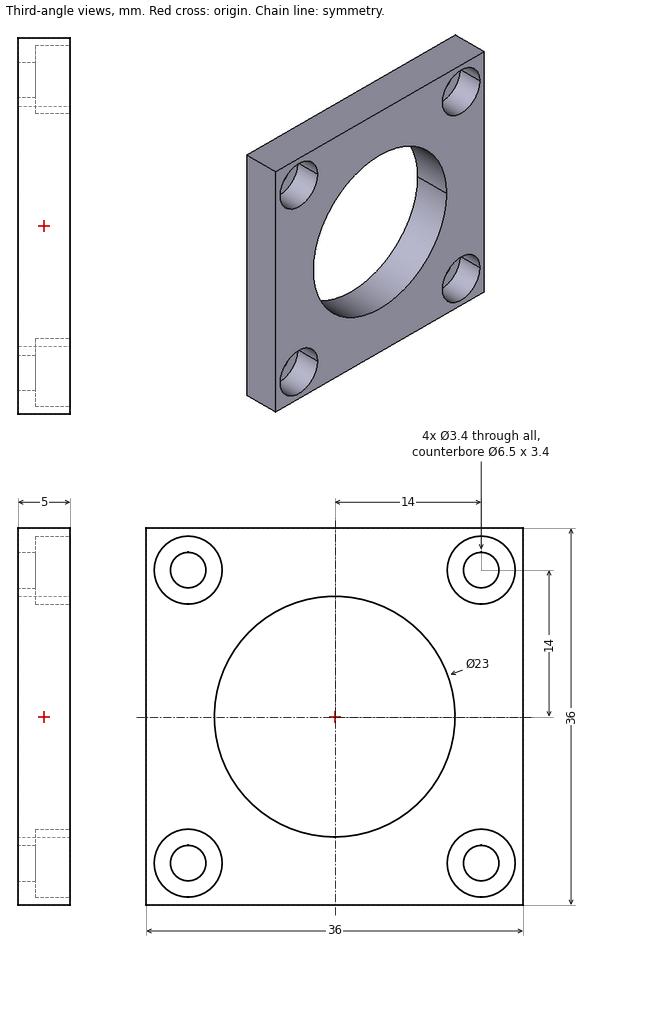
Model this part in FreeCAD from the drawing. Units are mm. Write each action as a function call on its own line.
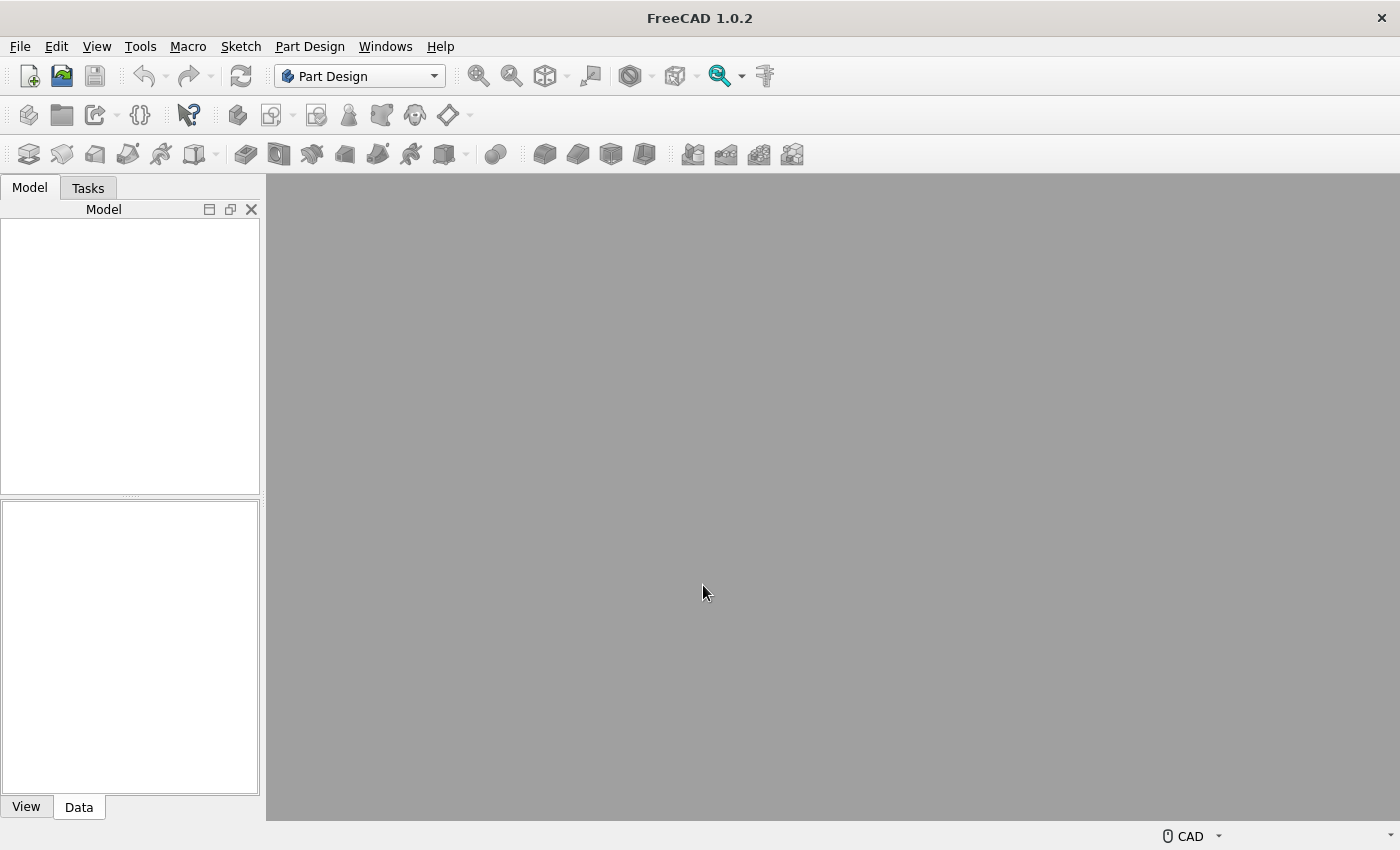
click(29, 76)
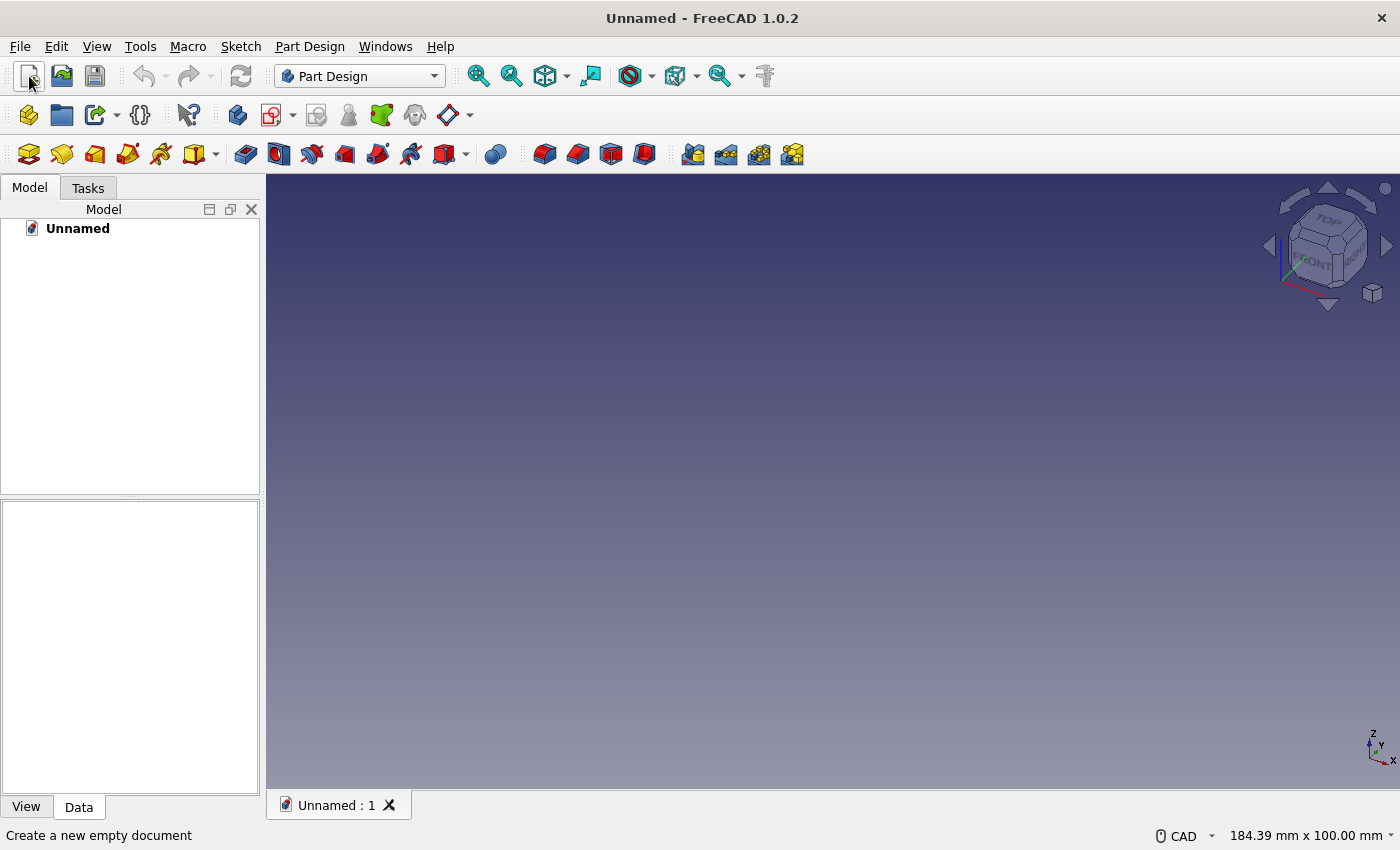
click(270, 116)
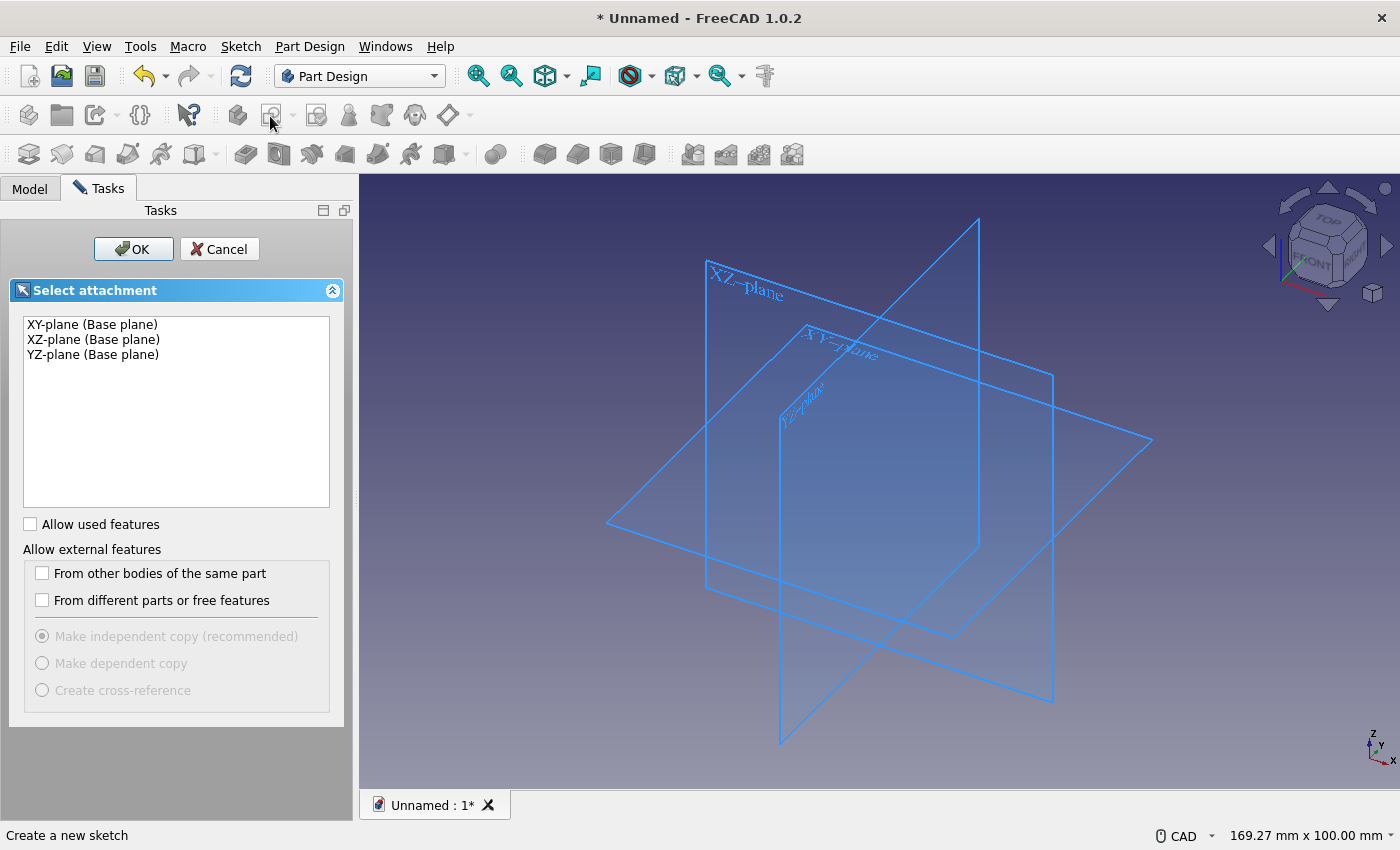
click(84, 354)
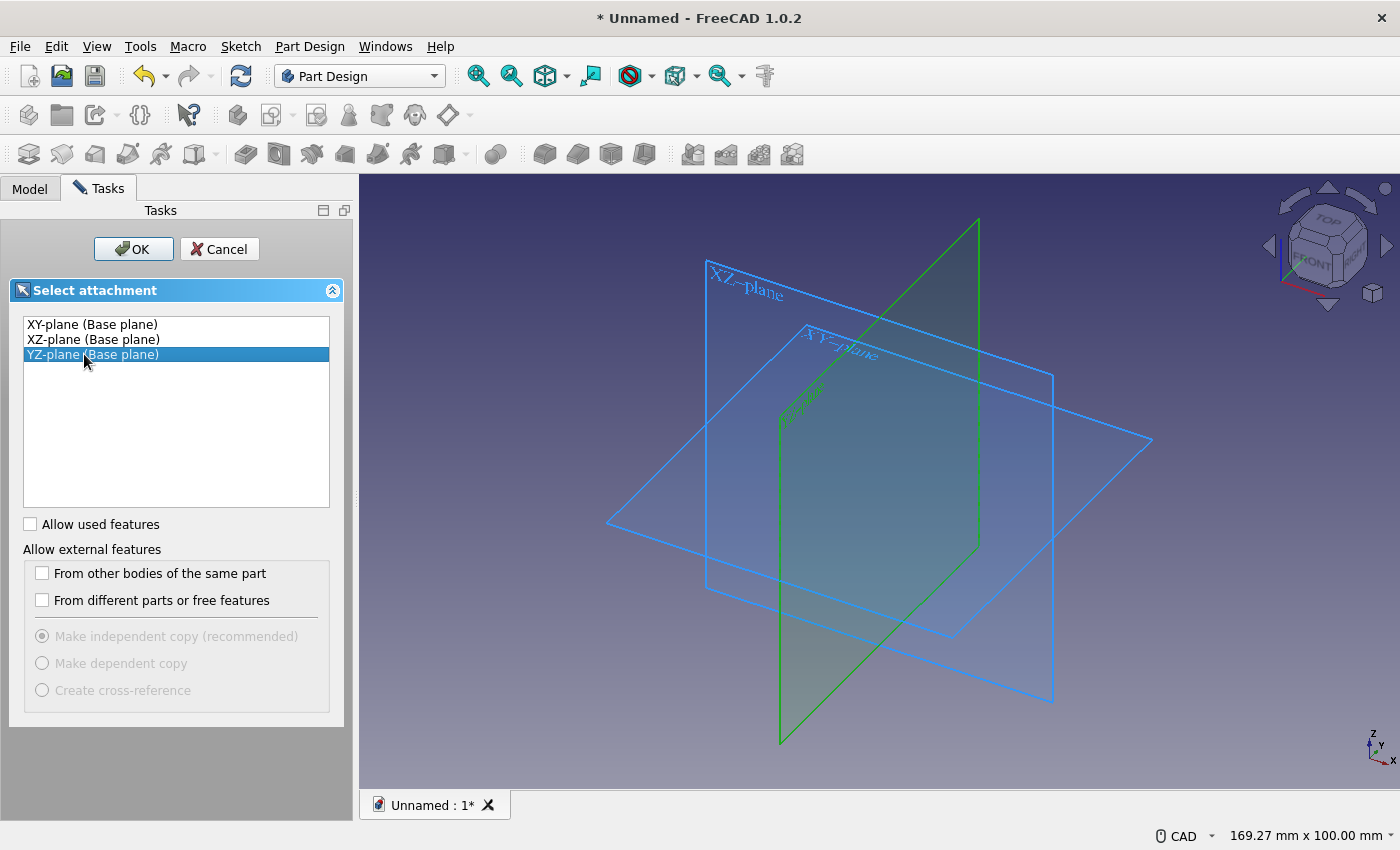
click(134, 249)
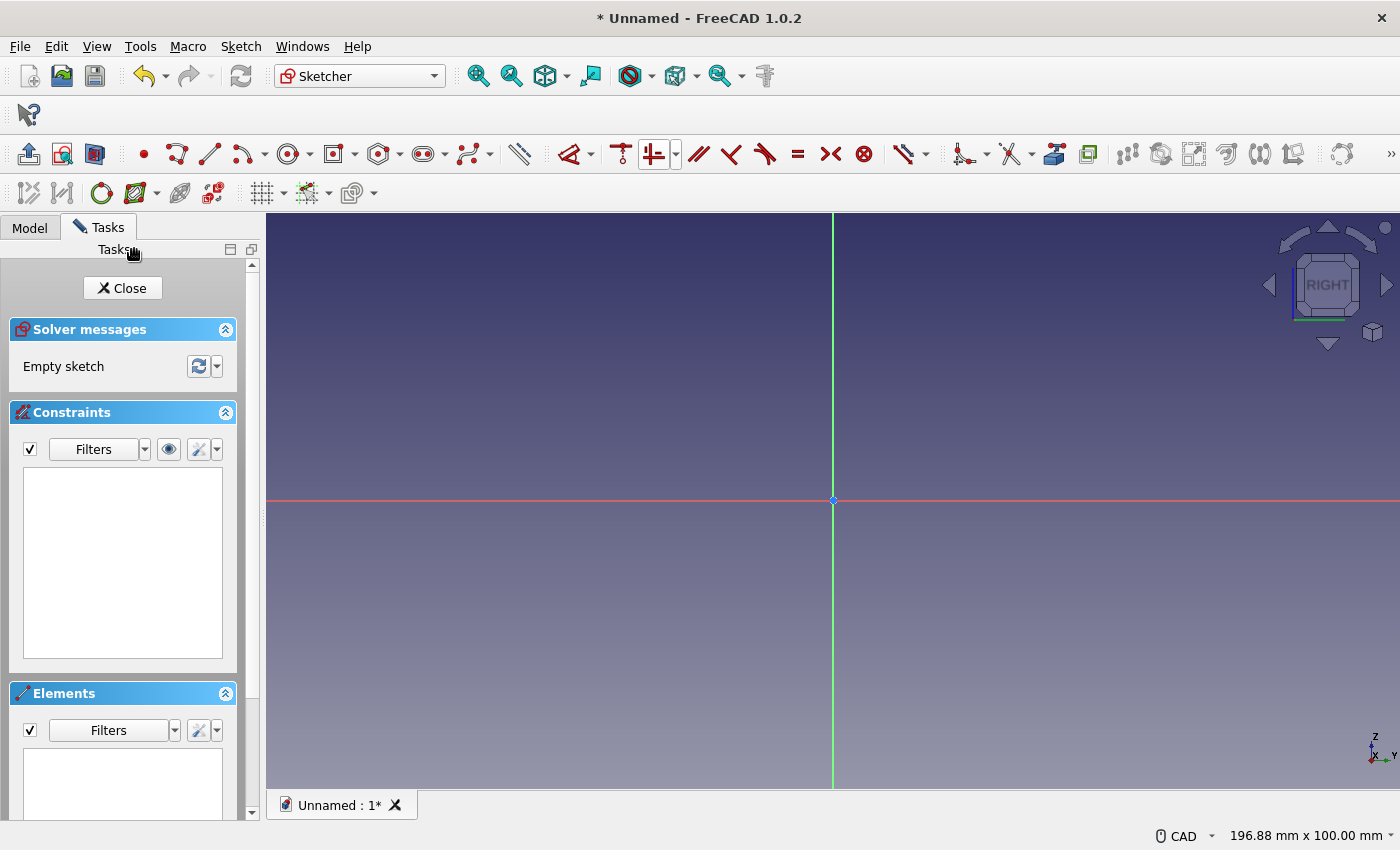
scroll(916, 501, up, 3)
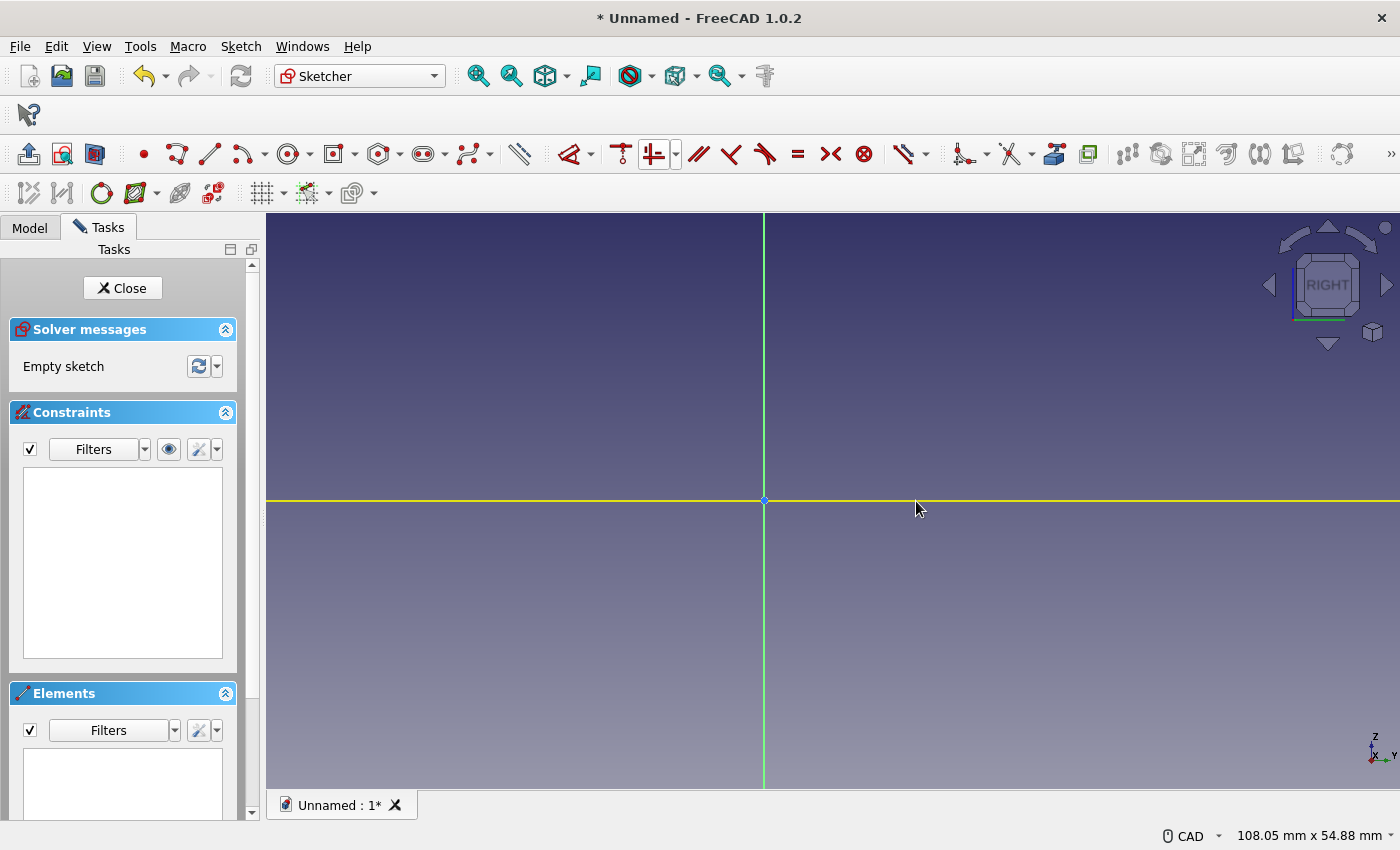
click(332, 154)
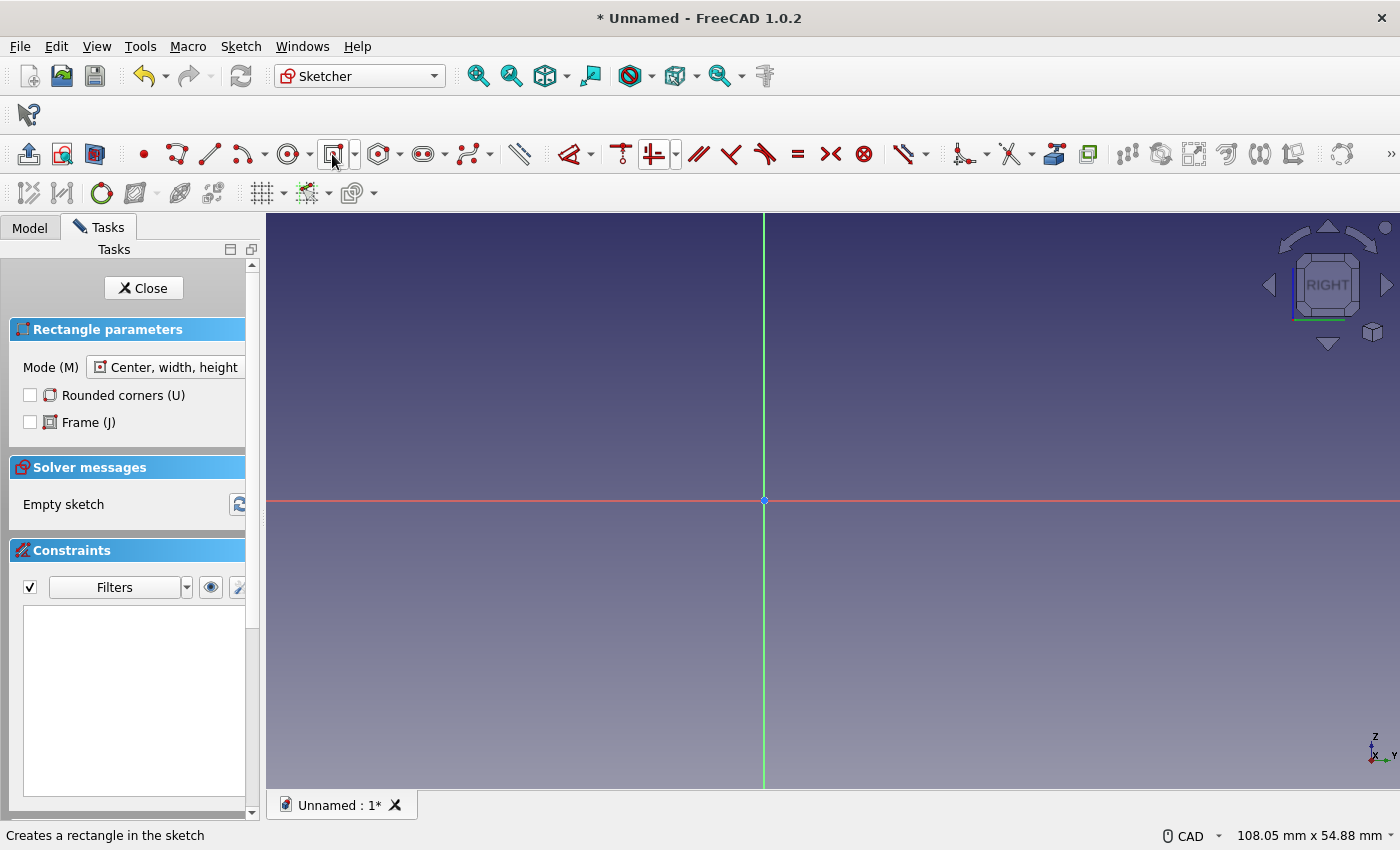
click(764, 501)
click(953, 312)
key(Escape)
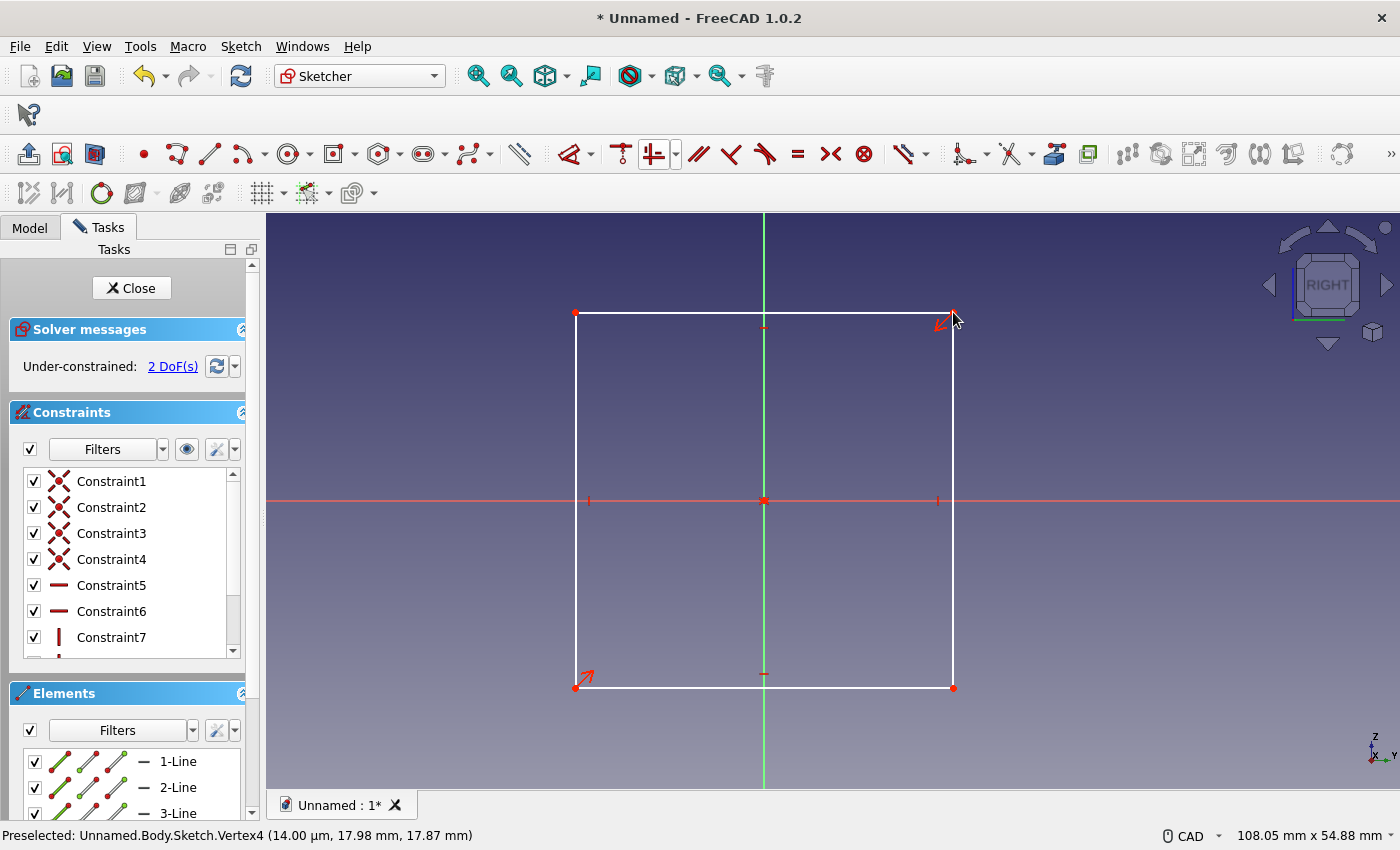
click(689, 688)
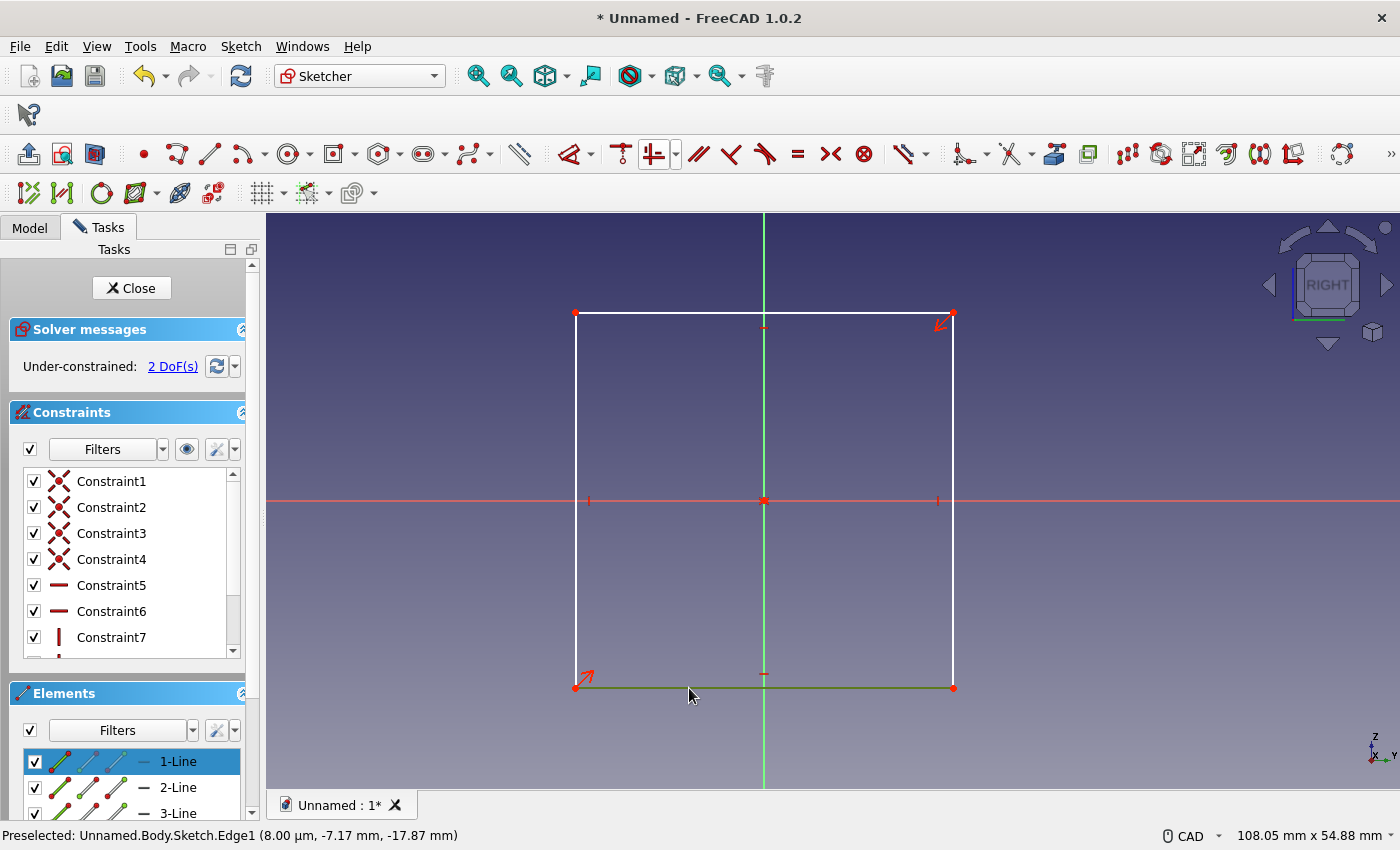
key(l)